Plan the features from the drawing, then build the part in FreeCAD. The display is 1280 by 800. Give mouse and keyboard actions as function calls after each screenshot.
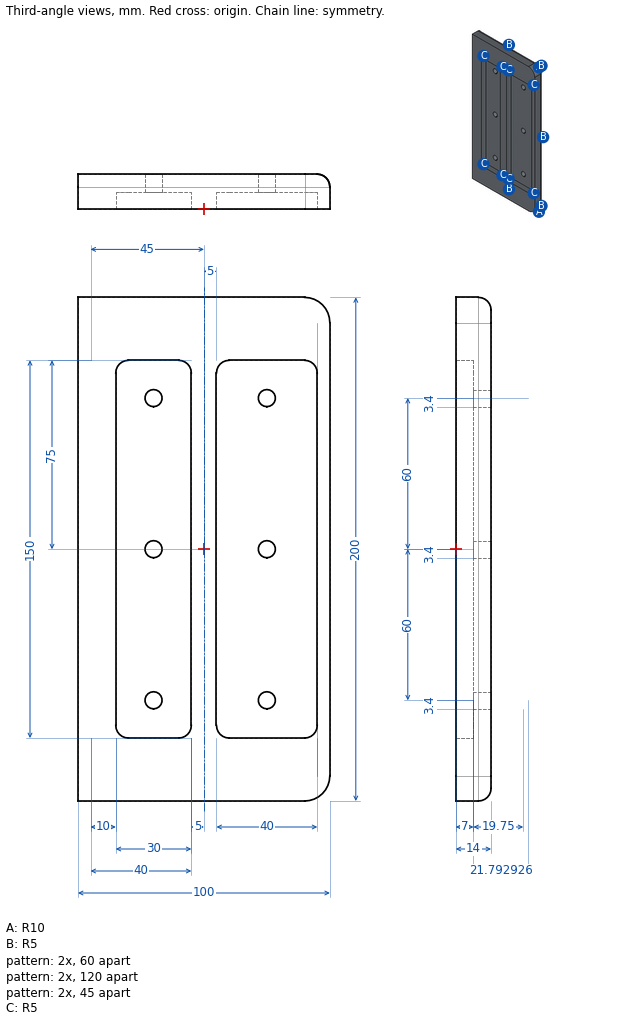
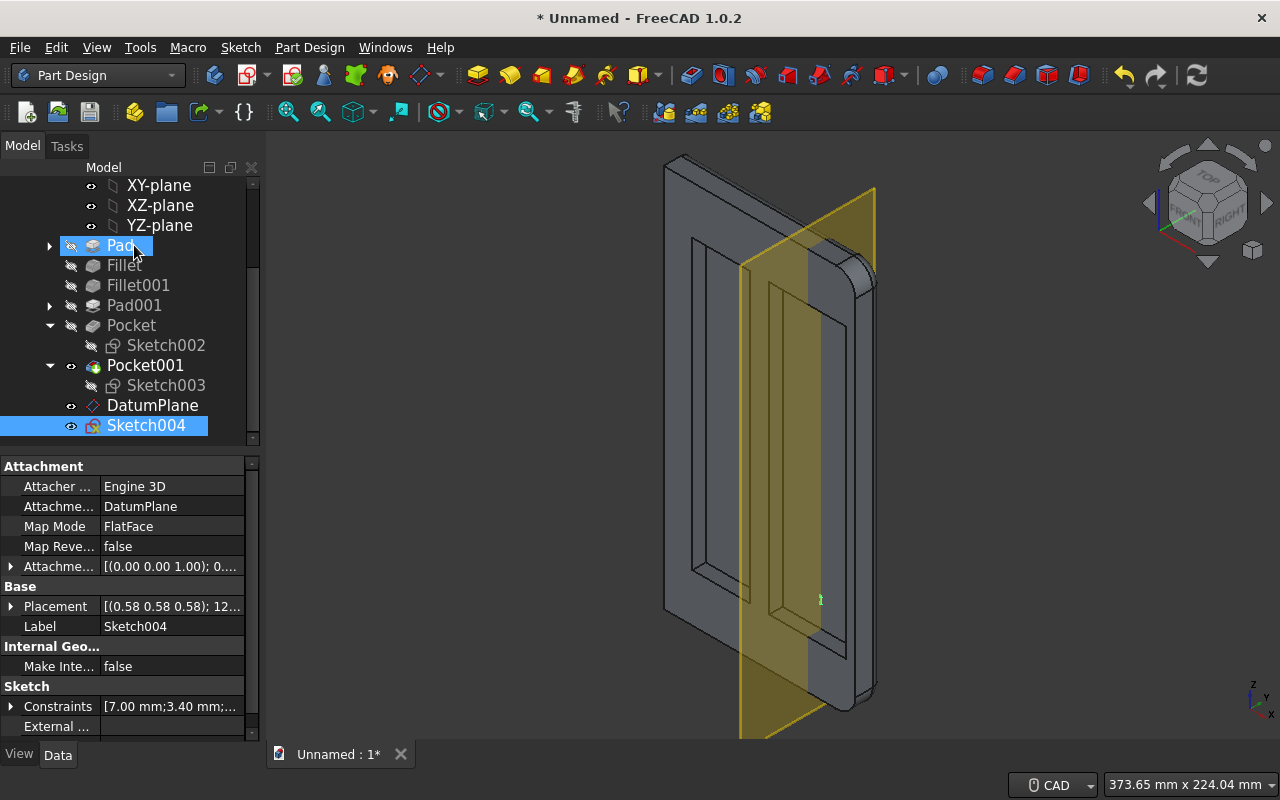
click(756, 76)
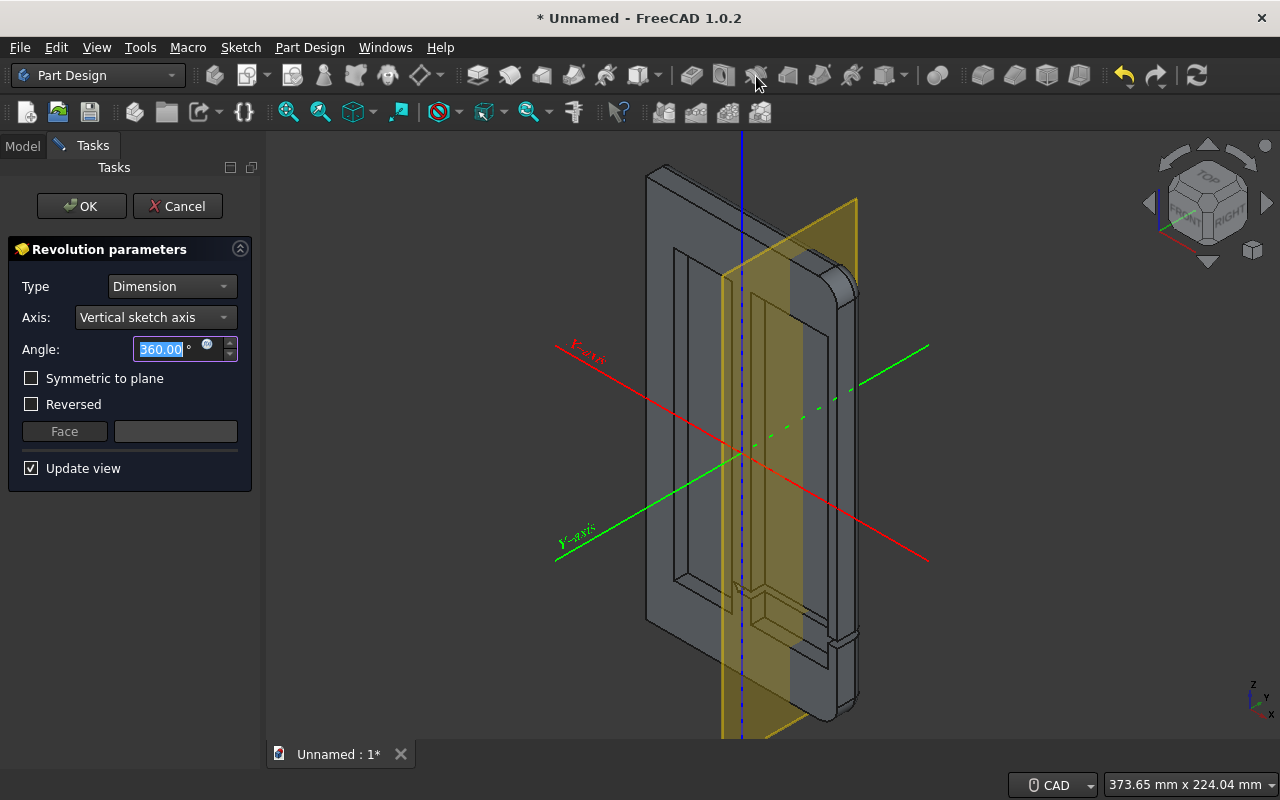
click(156, 318)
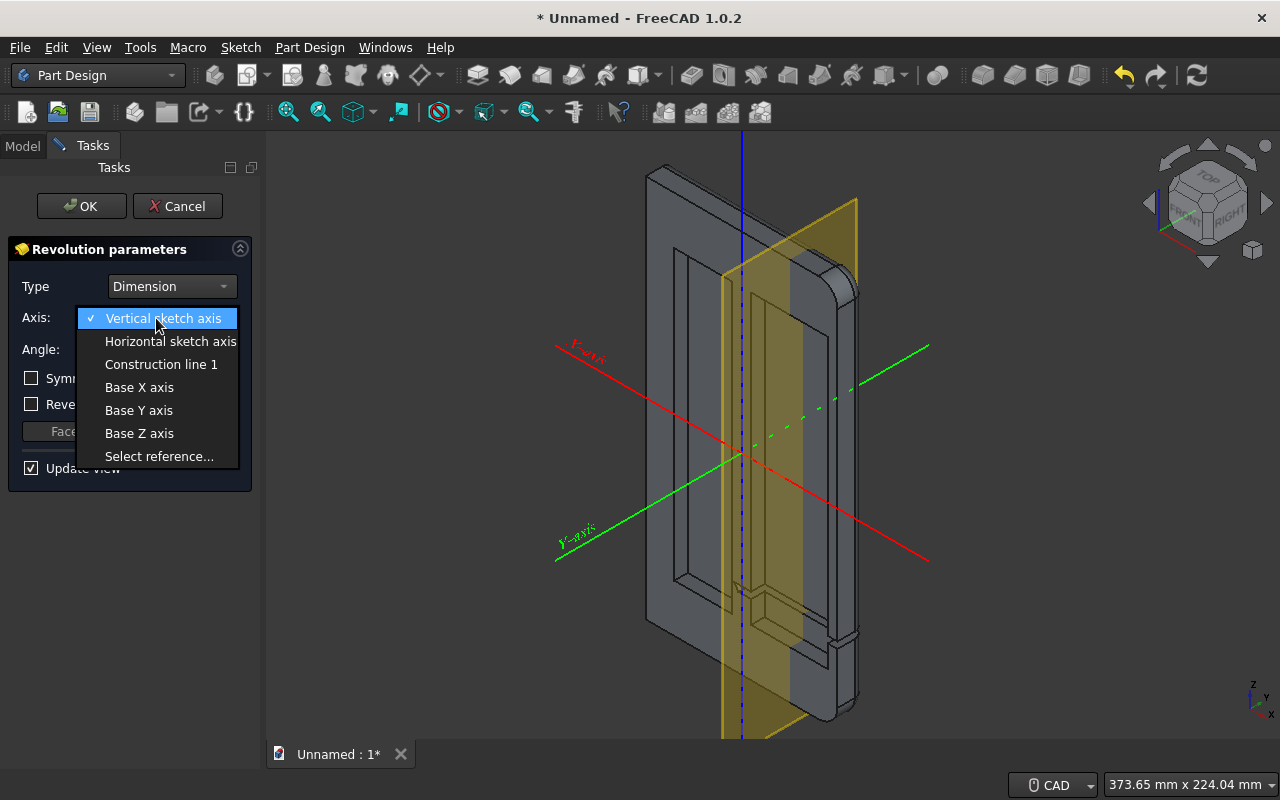
click(156, 364)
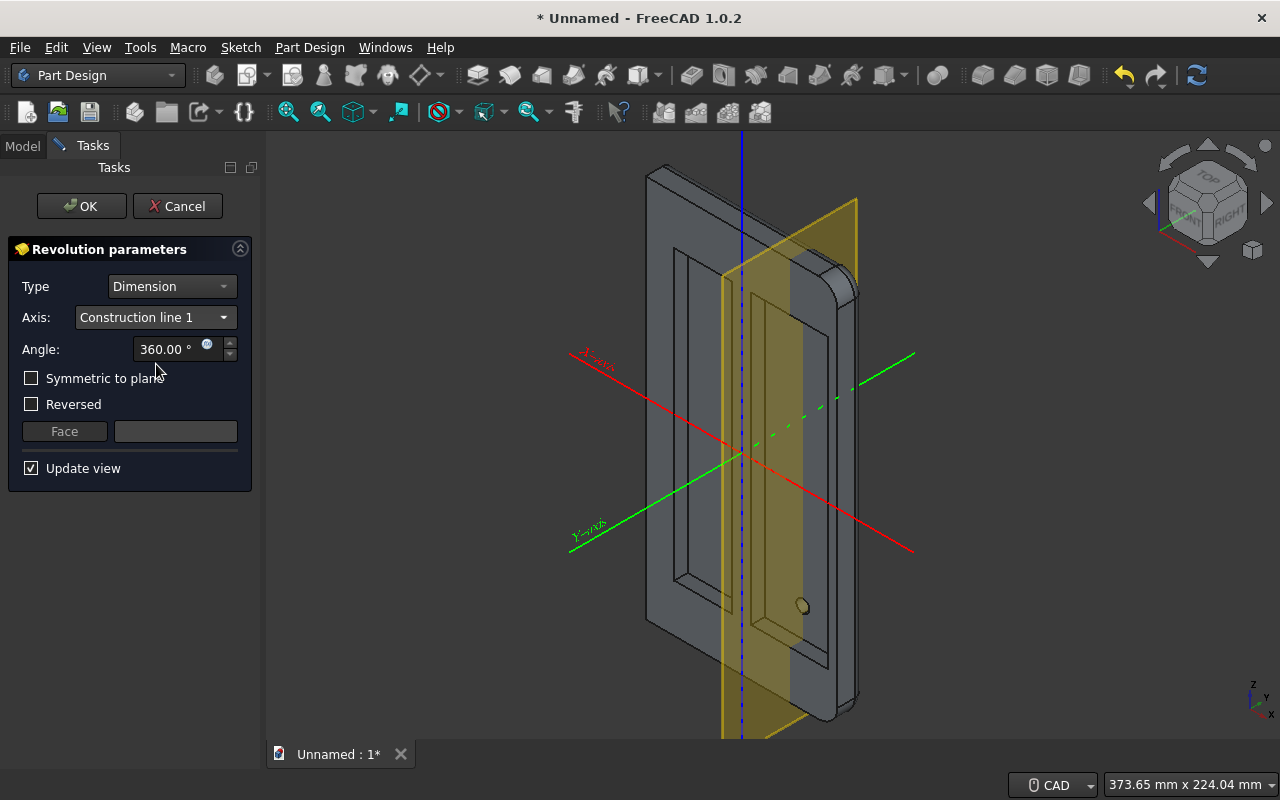
click(82, 206)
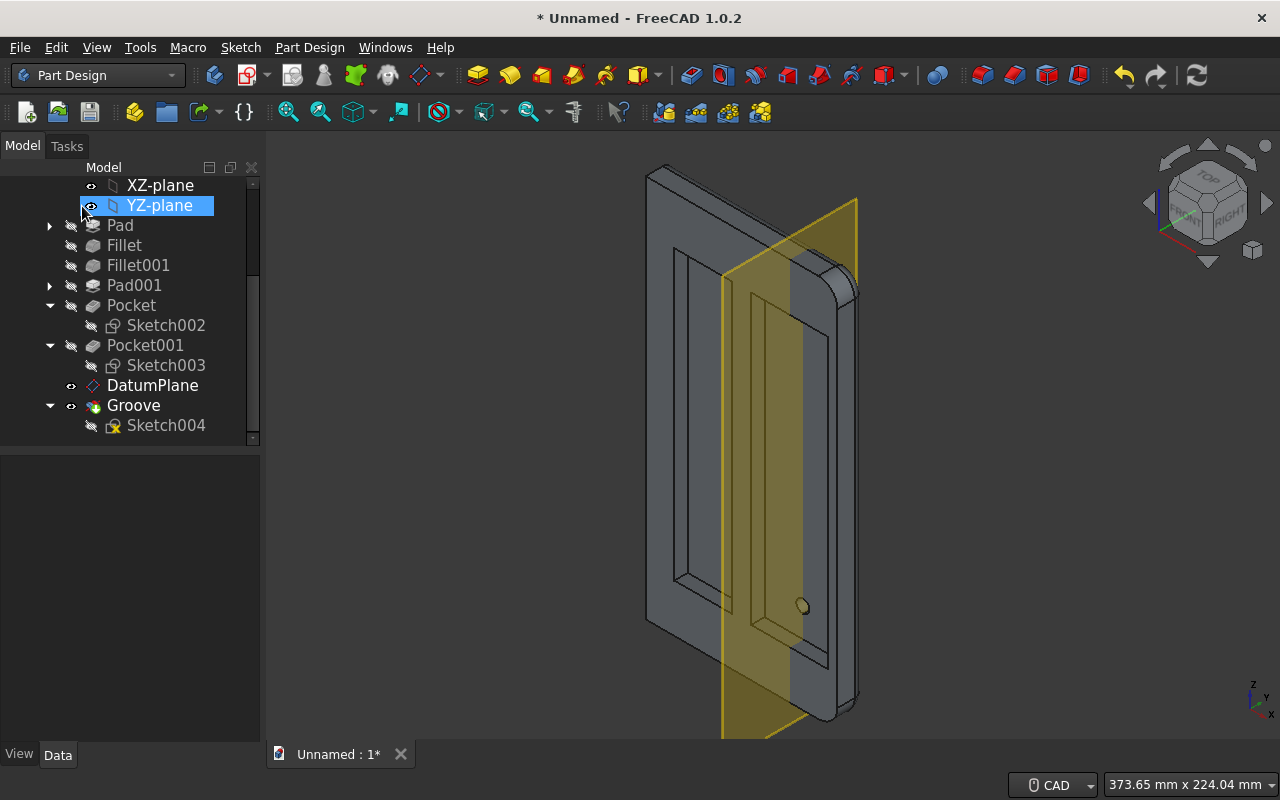
click(116, 386)
key(space)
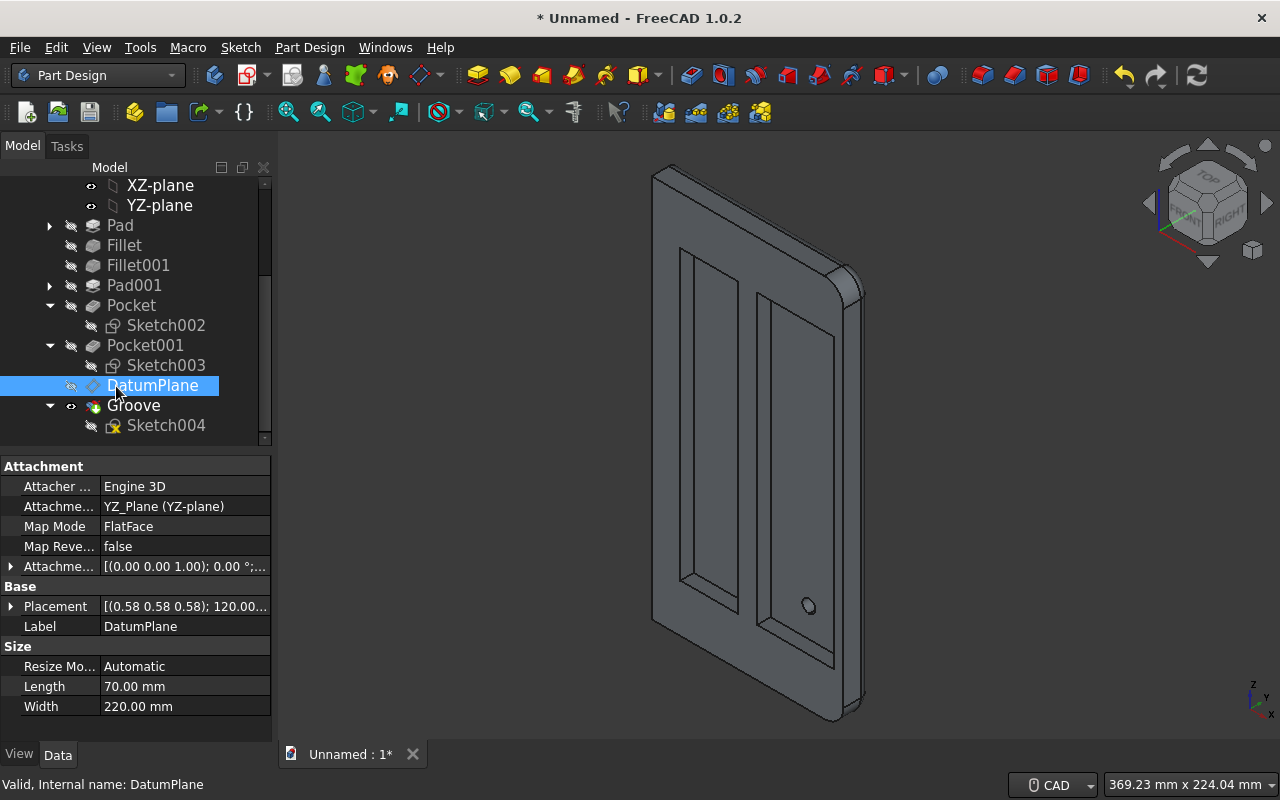
click(116, 406)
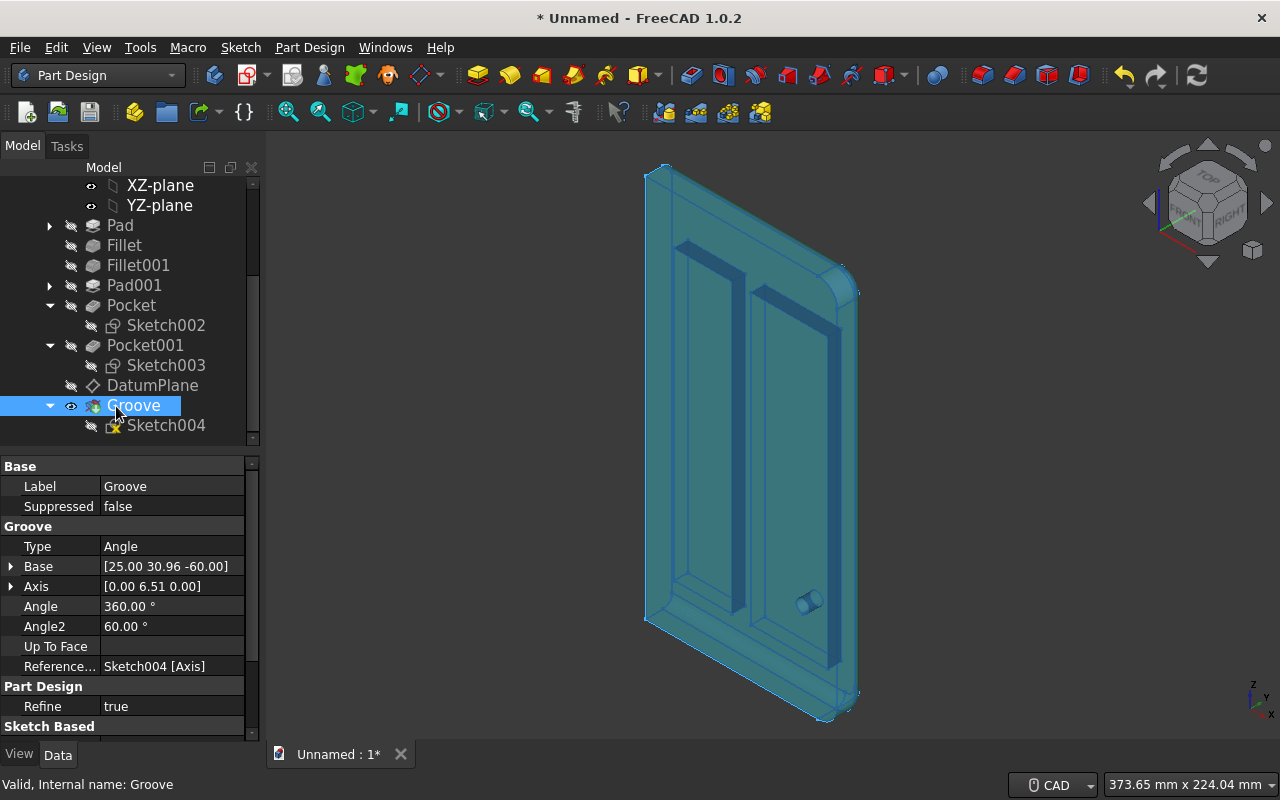
click(696, 112)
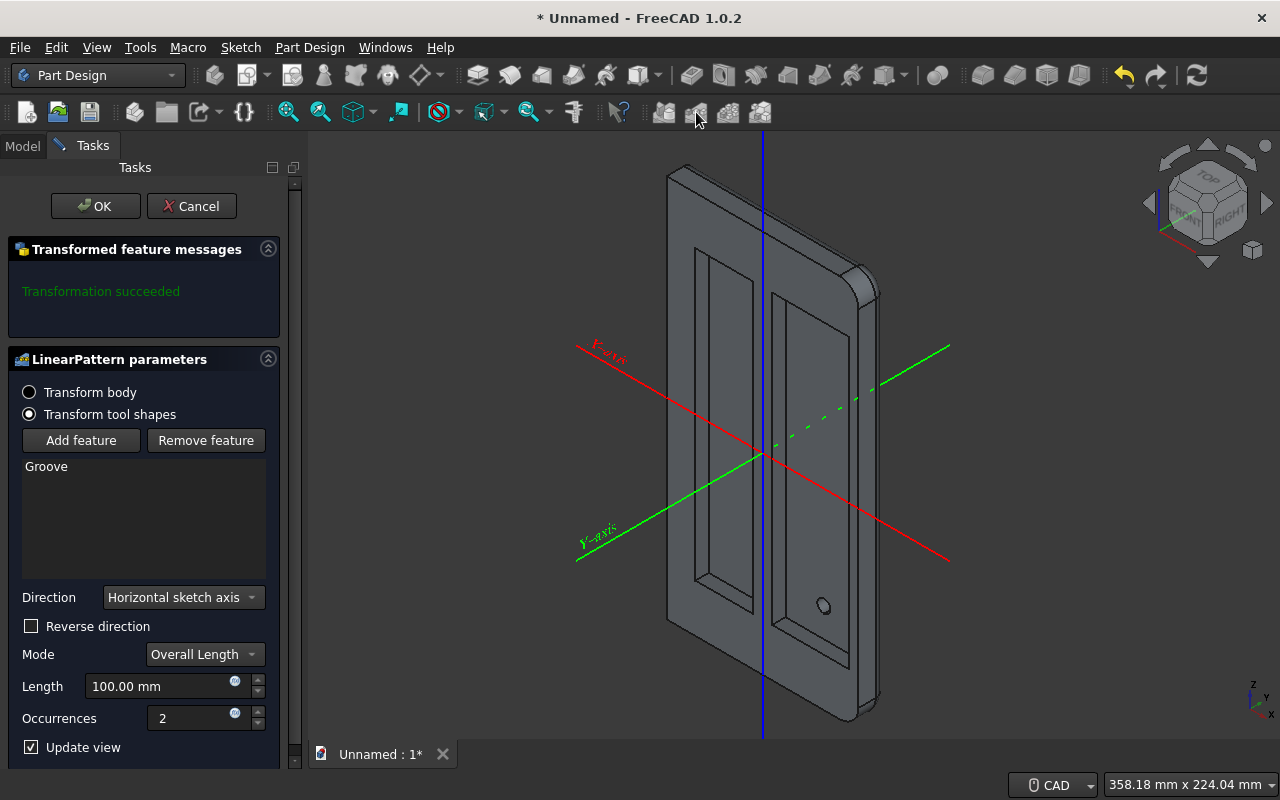
click(184, 598)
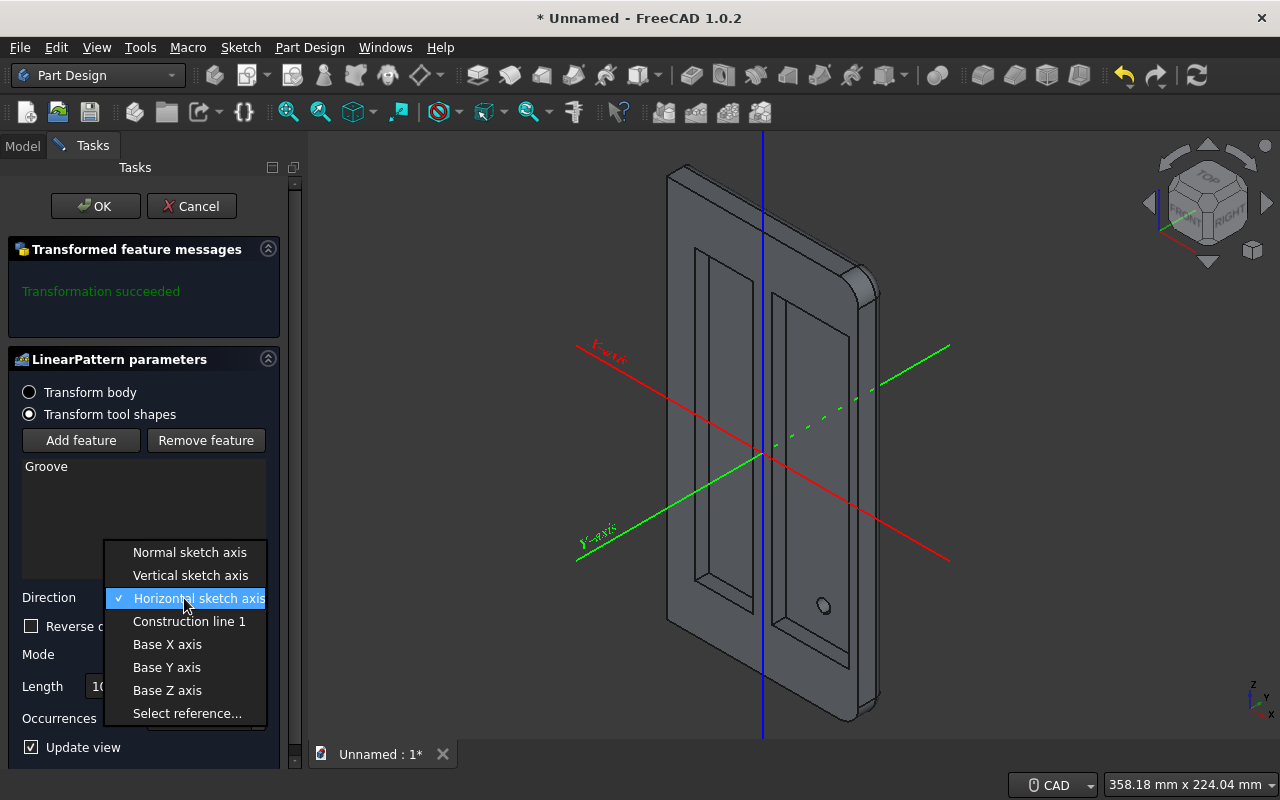
click(184, 690)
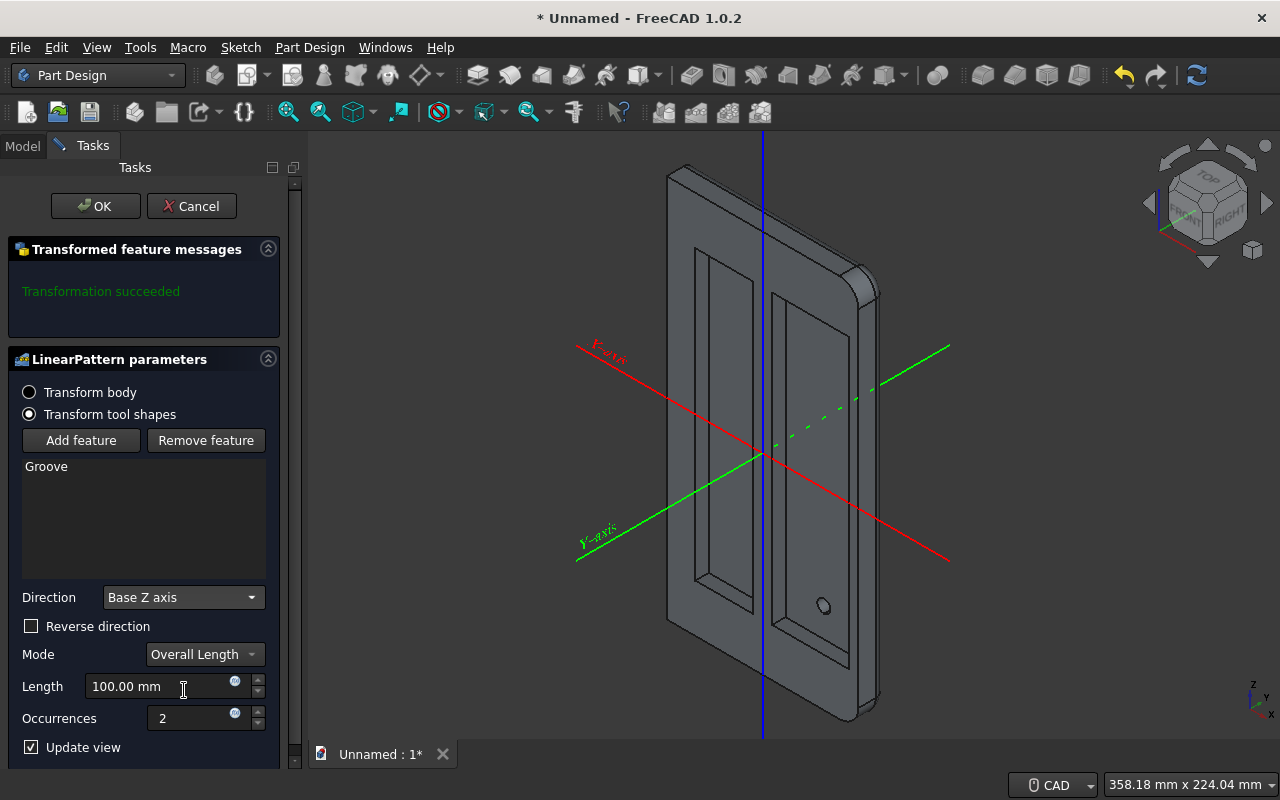
click(206, 654)